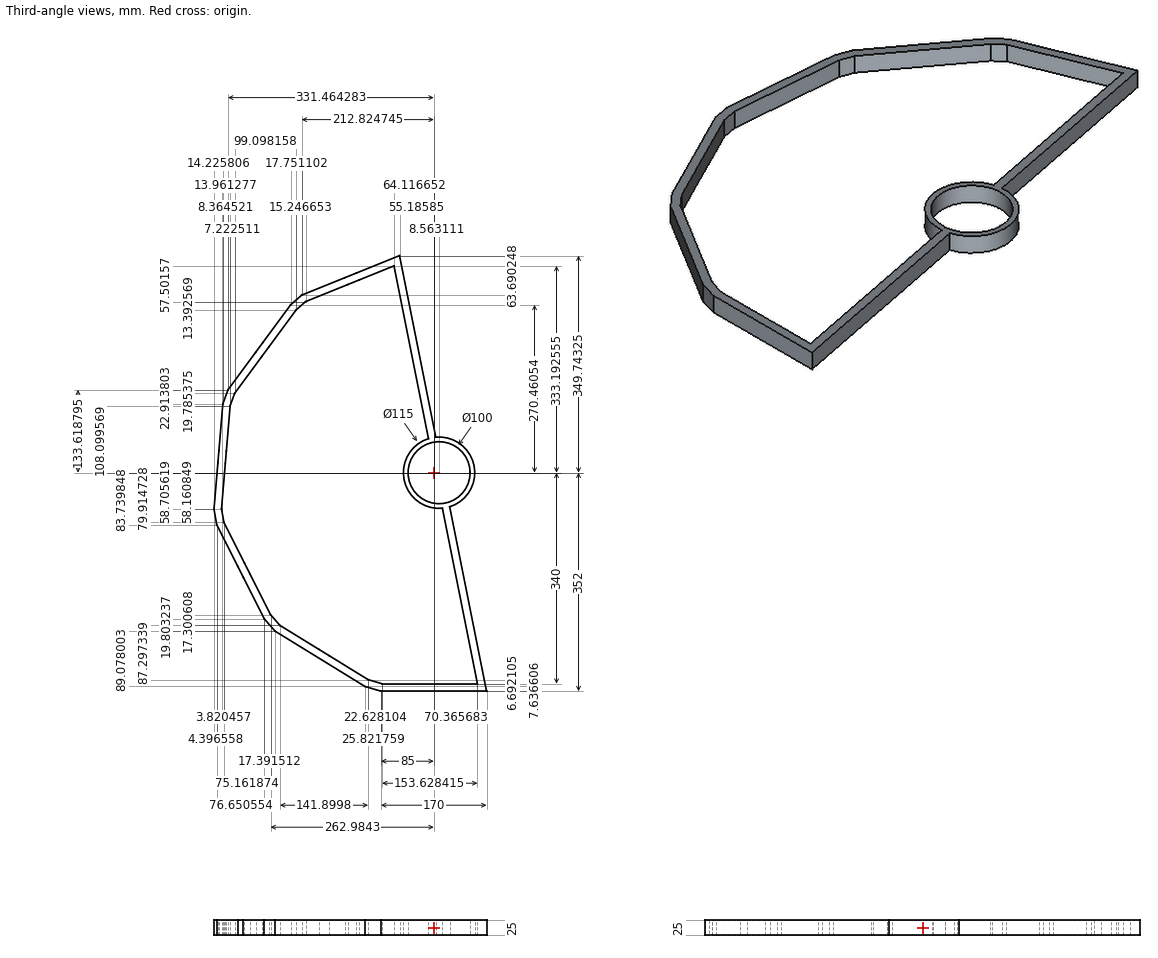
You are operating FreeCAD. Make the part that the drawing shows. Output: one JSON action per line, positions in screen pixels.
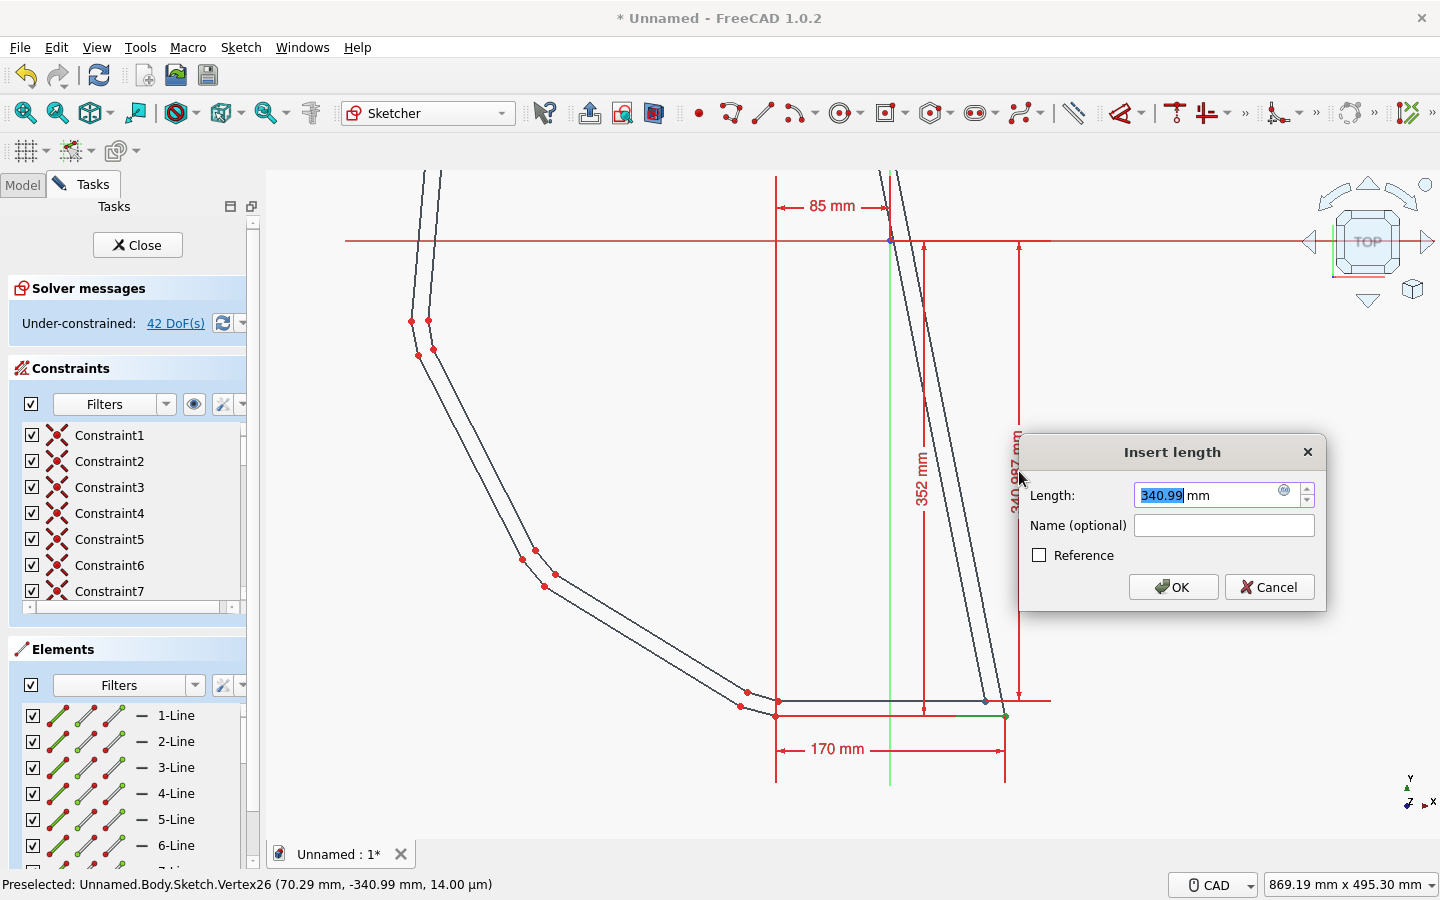
{"action": "type", "text": "340"}
{"action": "key", "text": "Return"}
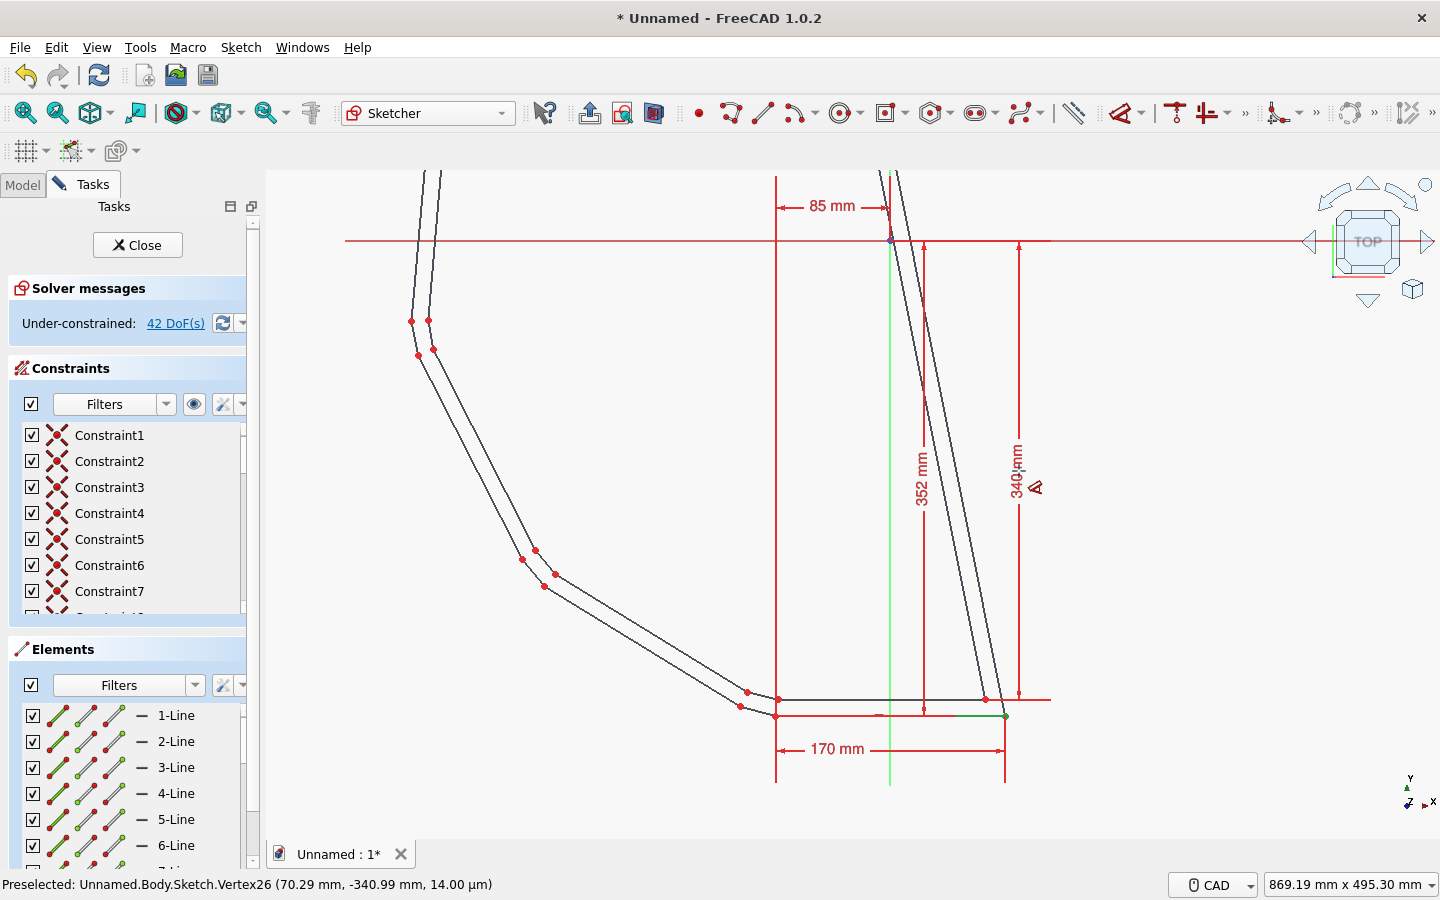
{"action": "scroll", "coordinate": [846, 719], "scroll_direction": "down", "scroll_amount": 4}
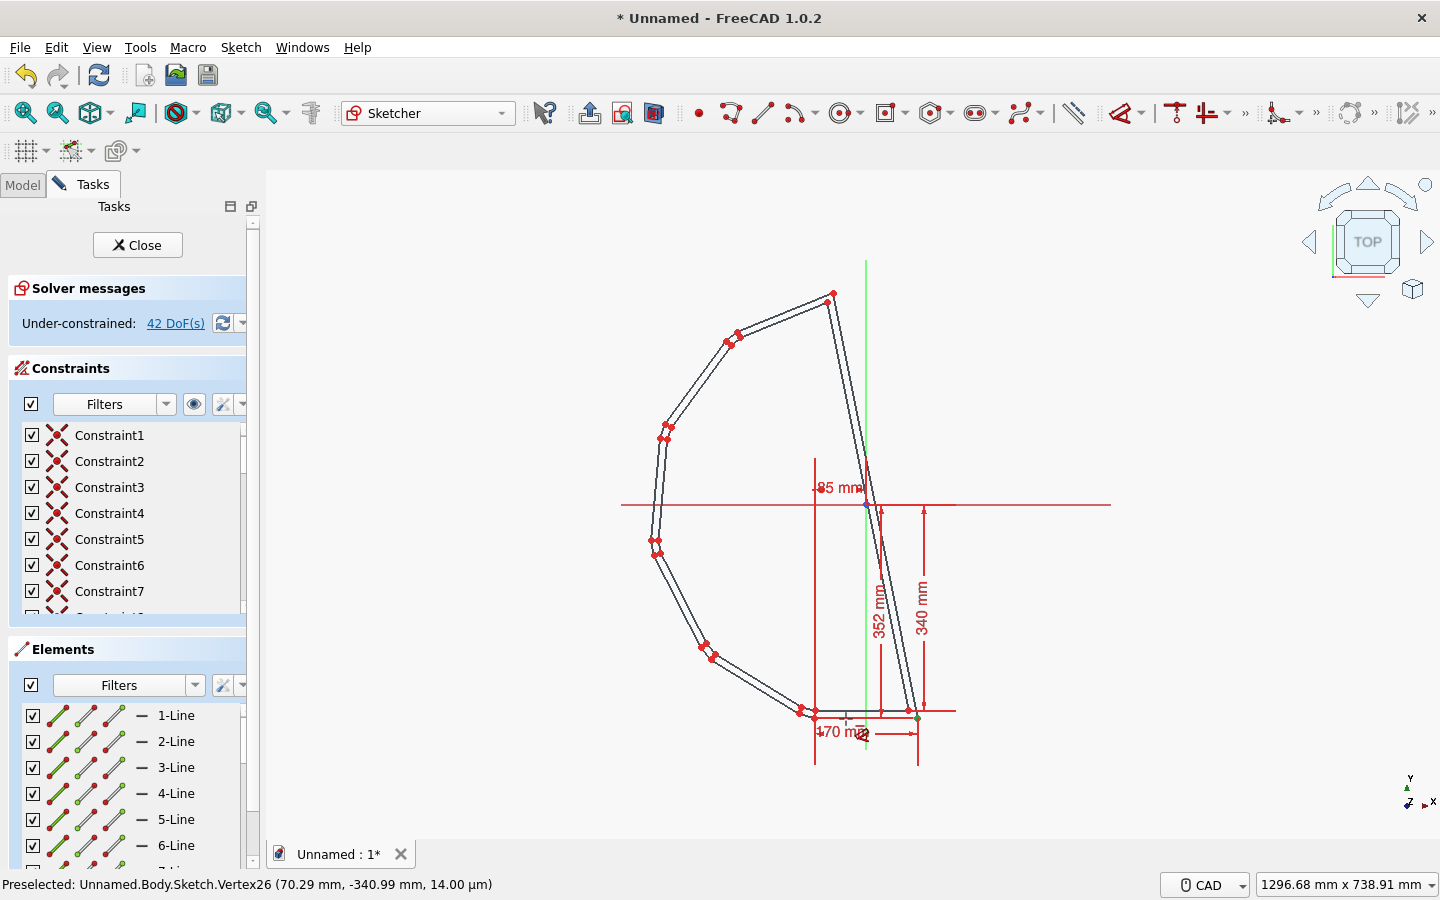
{"action": "left_click", "coordinate": [833, 293]}
{"action": "left_click", "coordinate": [850, 259]}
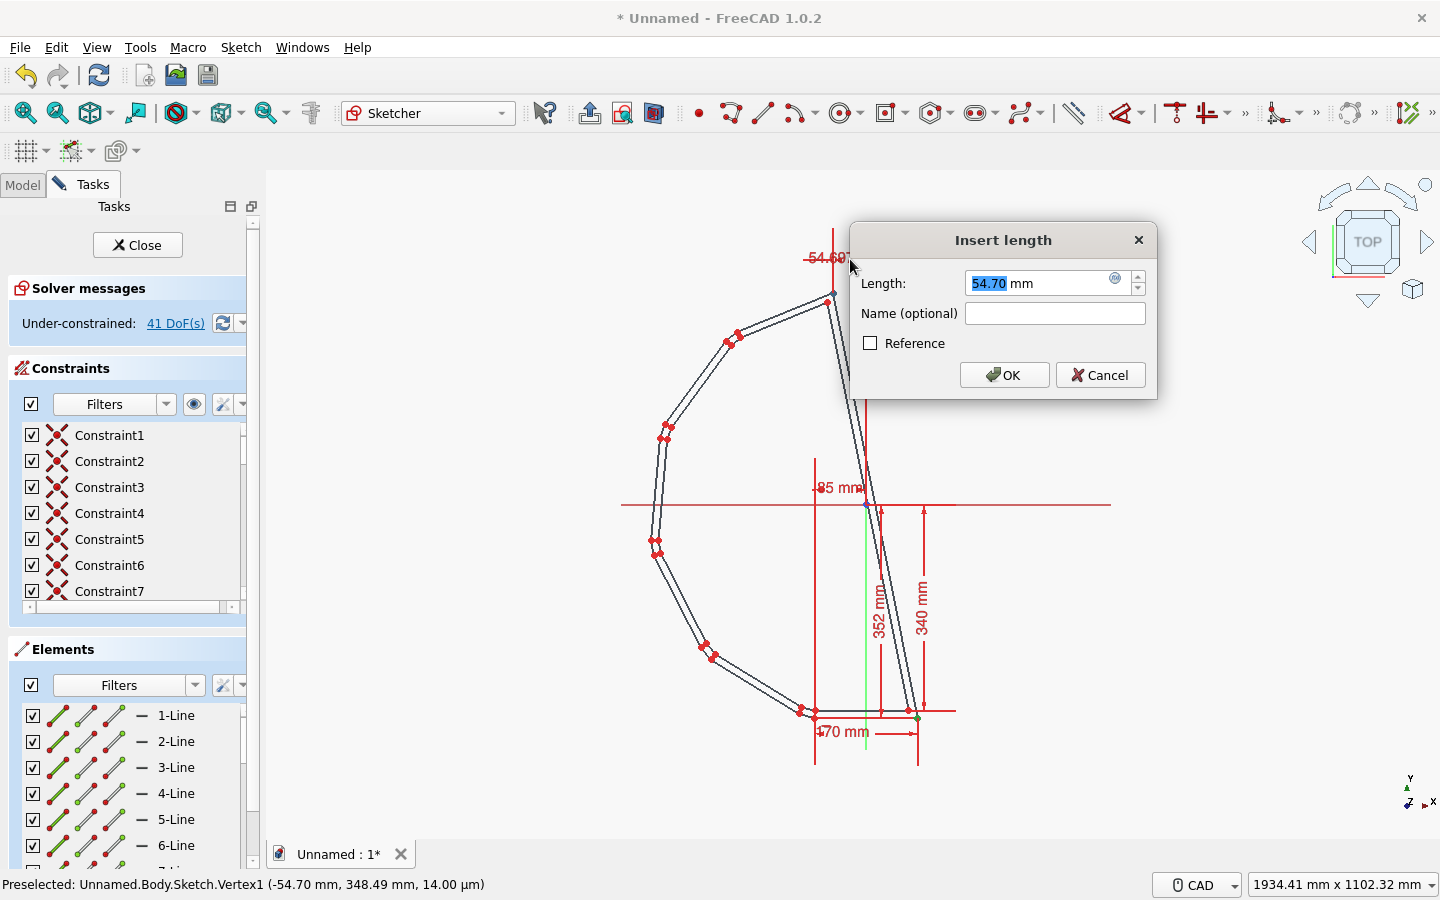
{"action": "type", "text": "55.18585"}
{"action": "key", "text": "Return"}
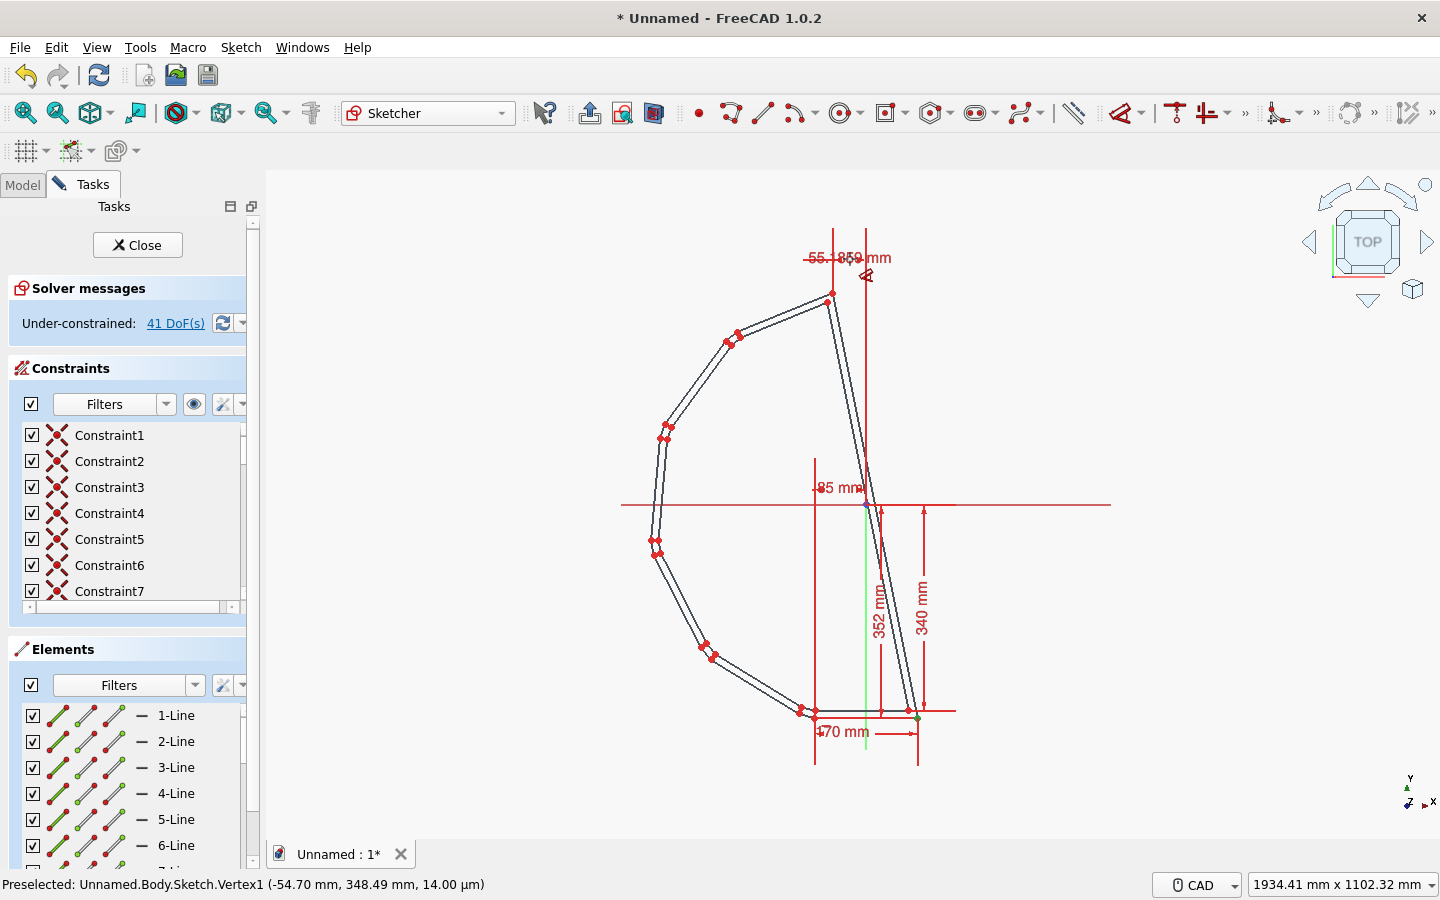
{"action": "scroll", "coordinate": [707, 644], "scroll_direction": "up", "scroll_amount": 3}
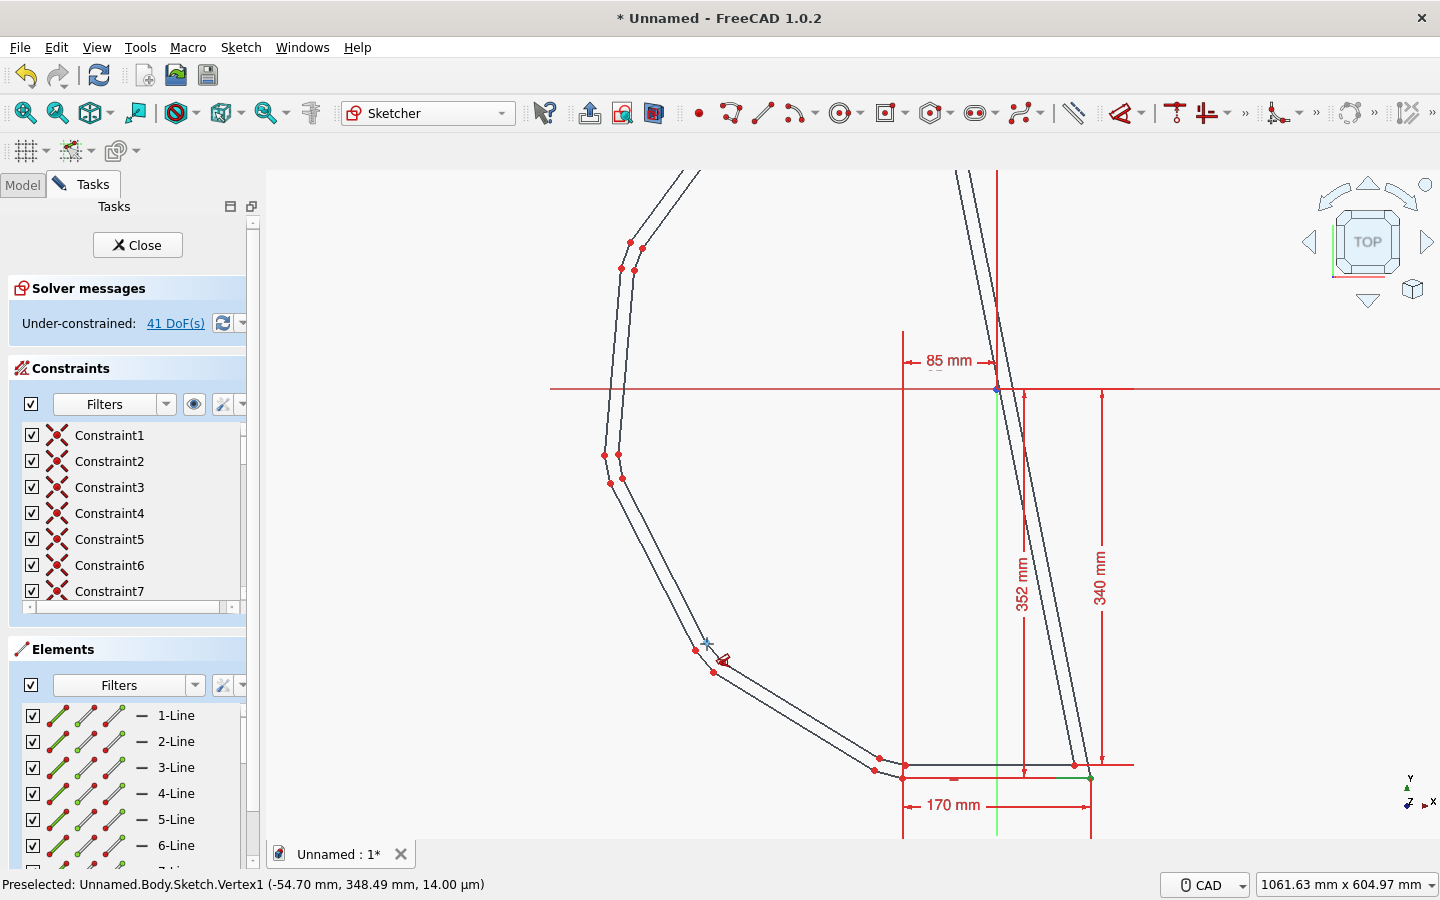
{"action": "left_click", "coordinate": [706, 643]}
{"action": "left_click", "coordinate": [851, 677]}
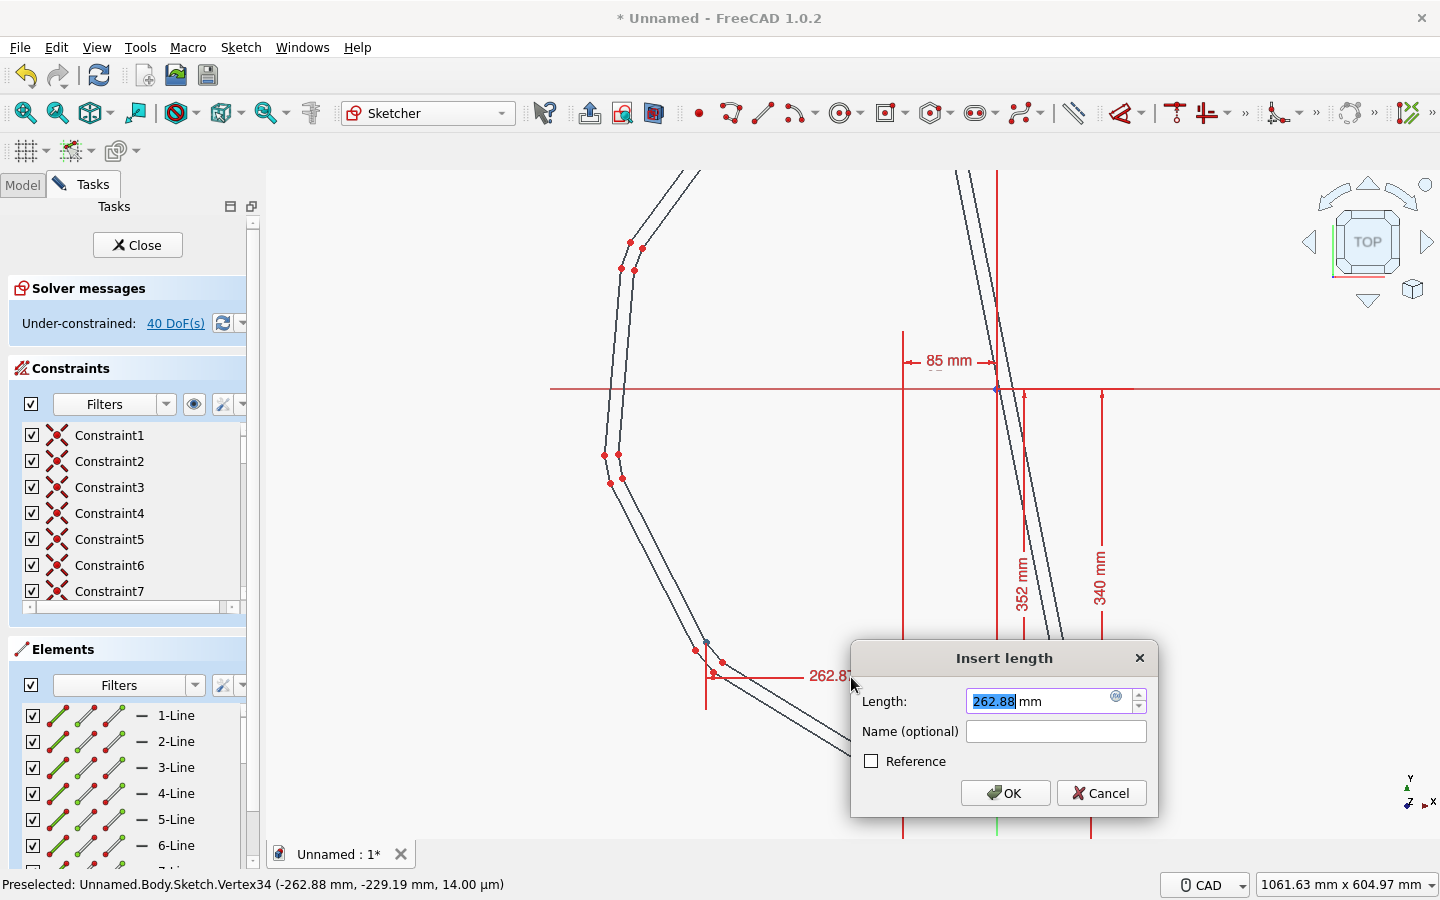
{"action": "type", "text": "262.9843"}
{"action": "key", "text": "Return"}